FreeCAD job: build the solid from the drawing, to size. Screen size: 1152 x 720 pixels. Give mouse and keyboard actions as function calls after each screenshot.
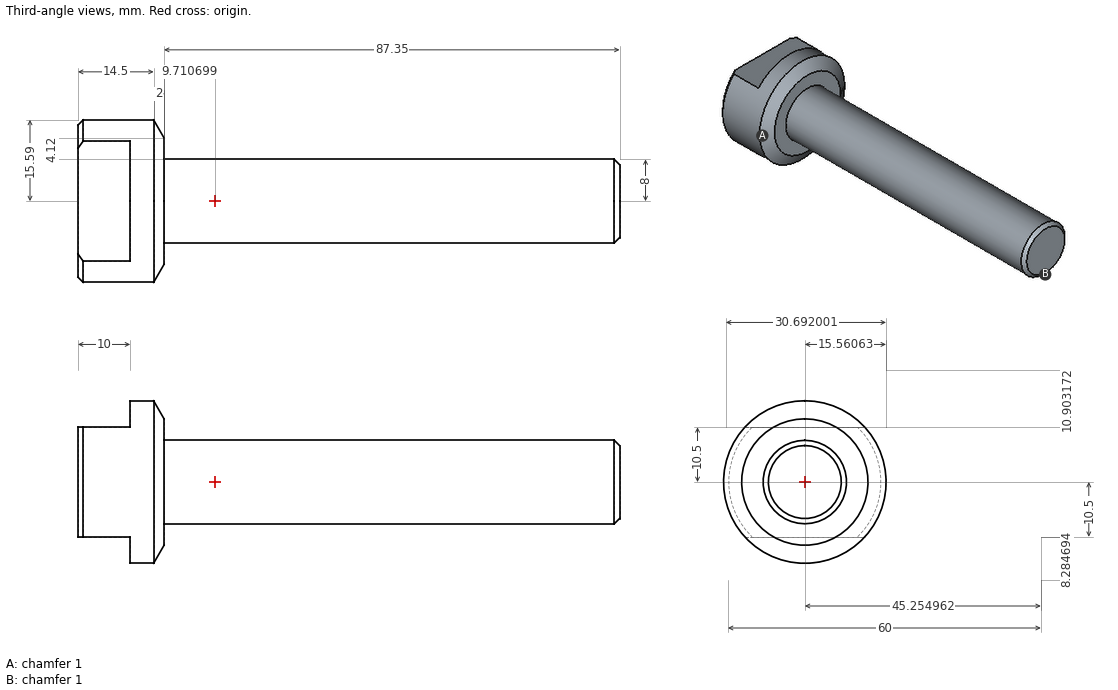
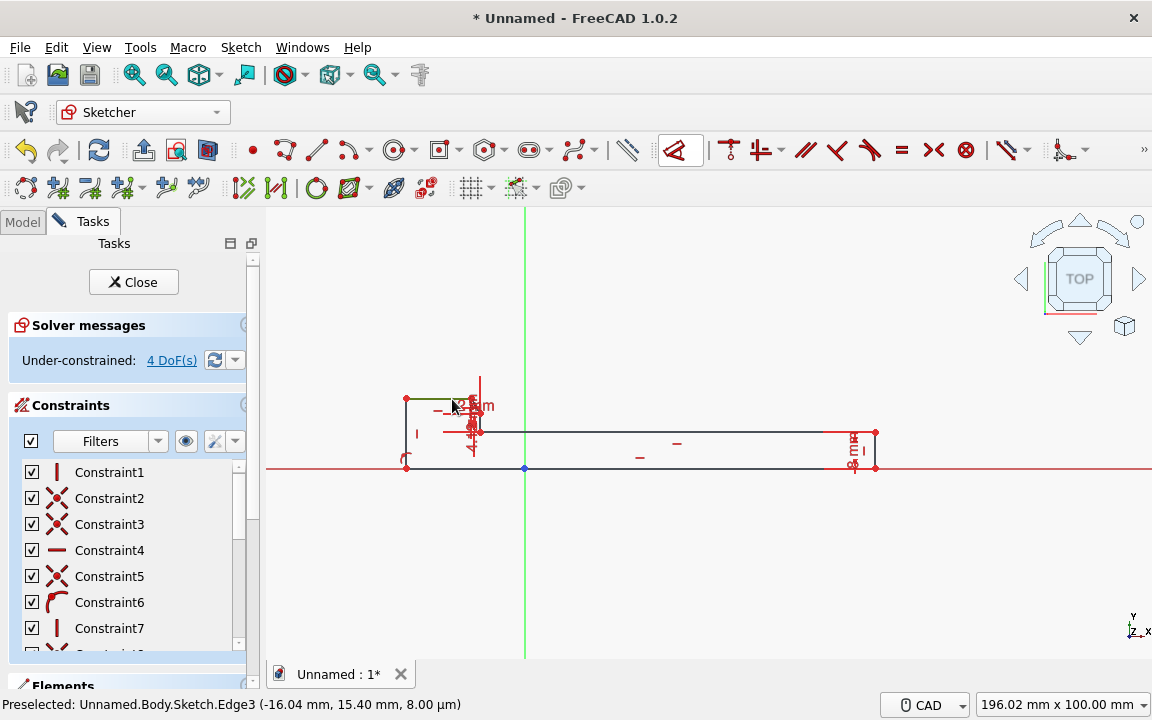
click(698, 150)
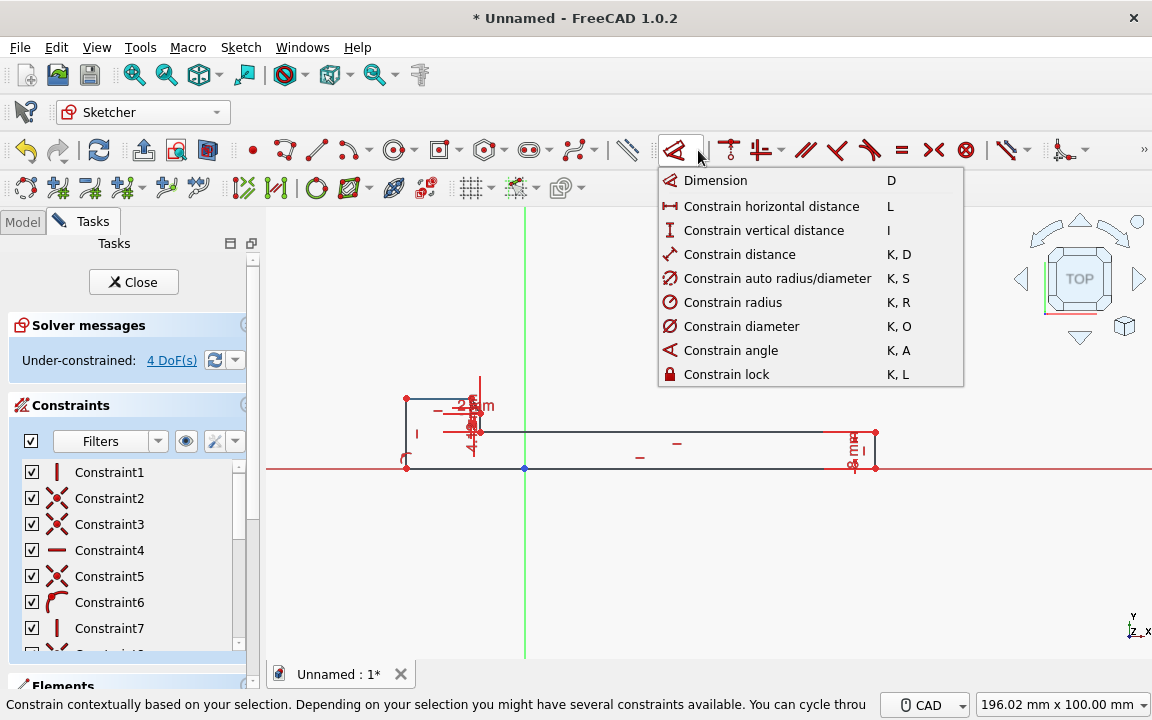
click(811, 206)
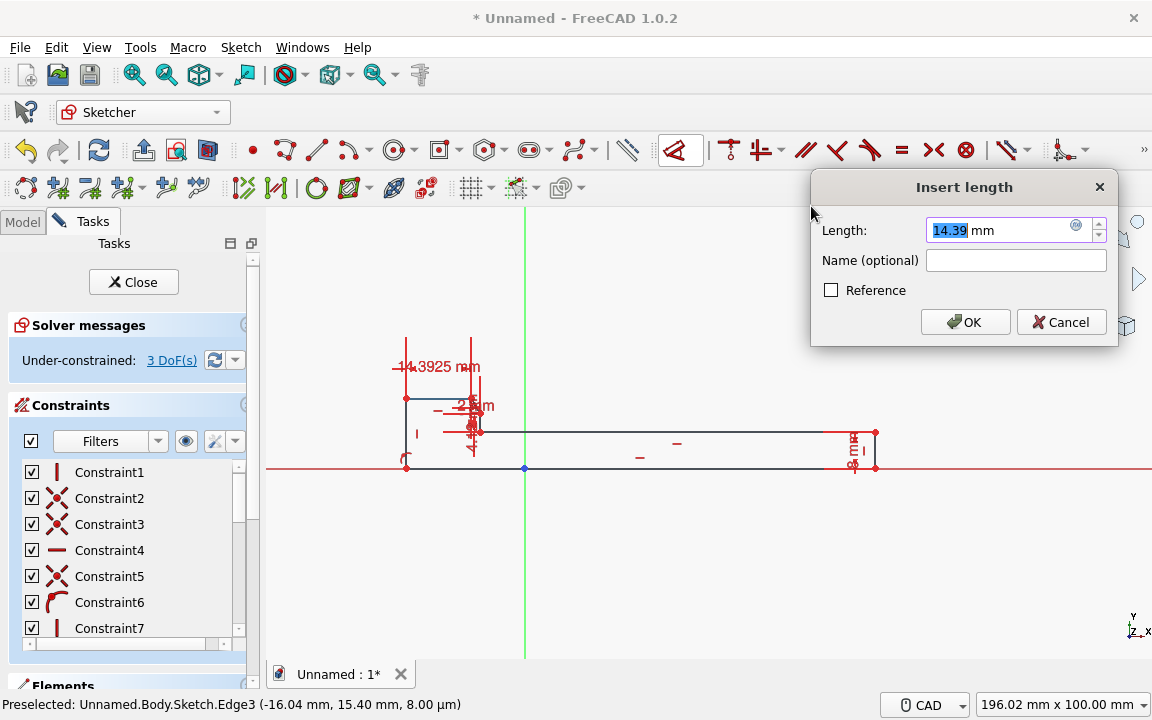
text(14.5)
key(Return)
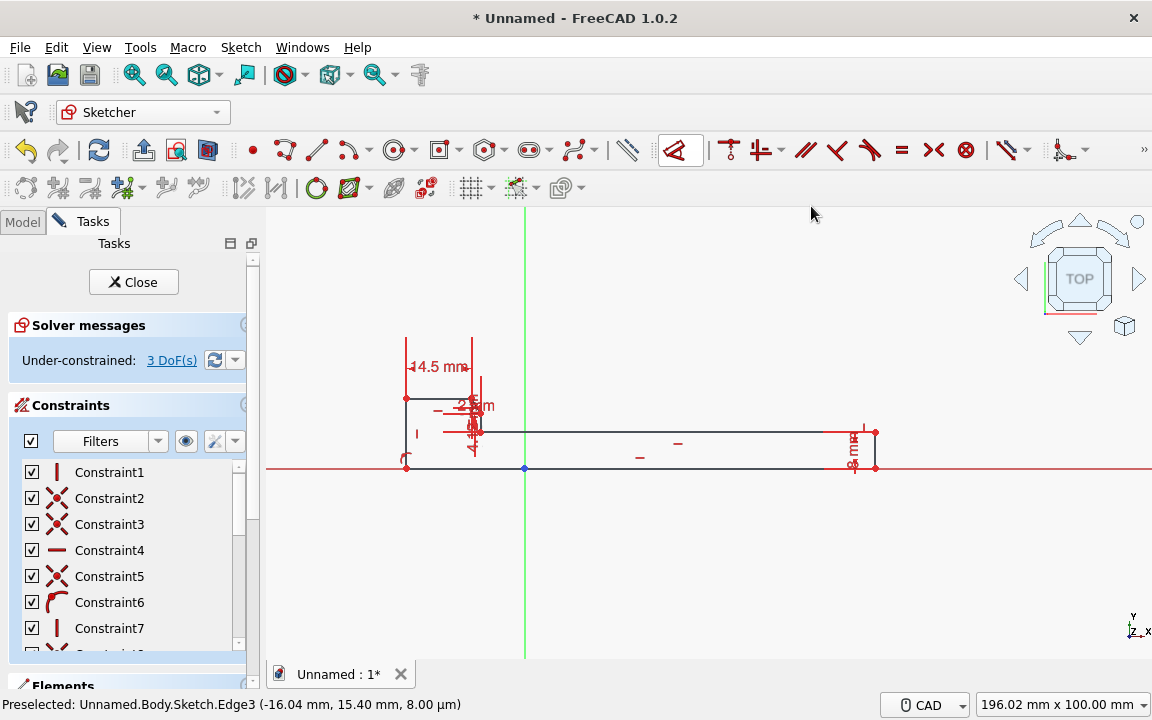
click(406, 420)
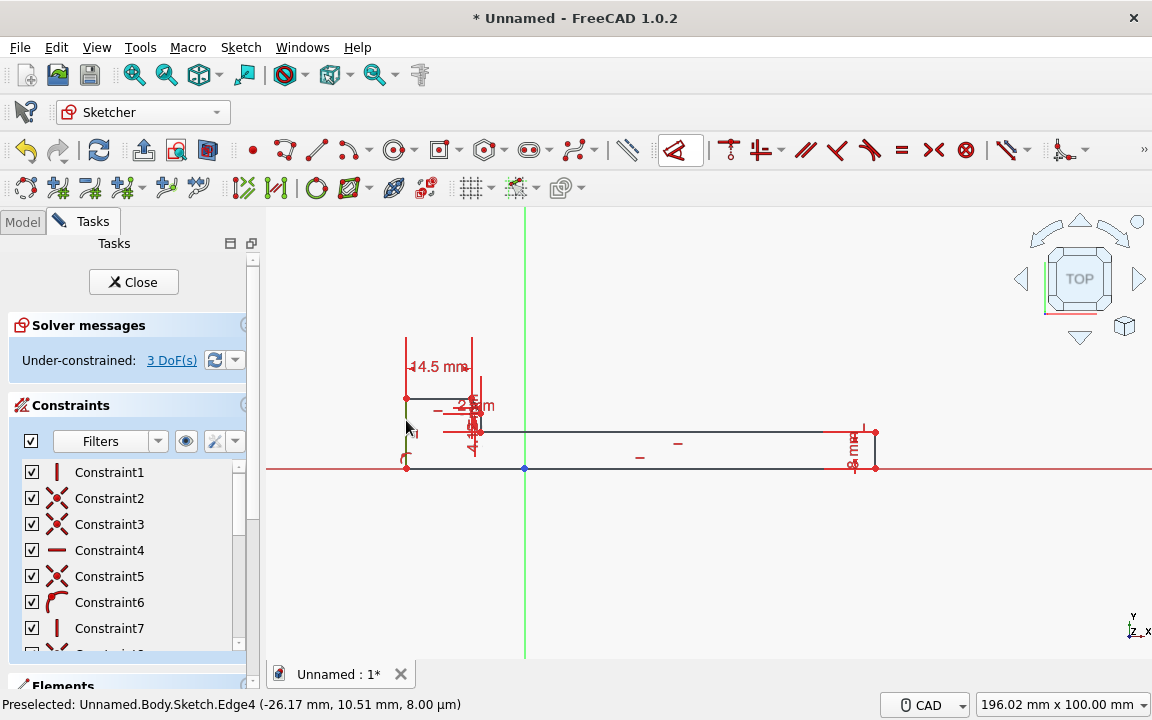
click(698, 150)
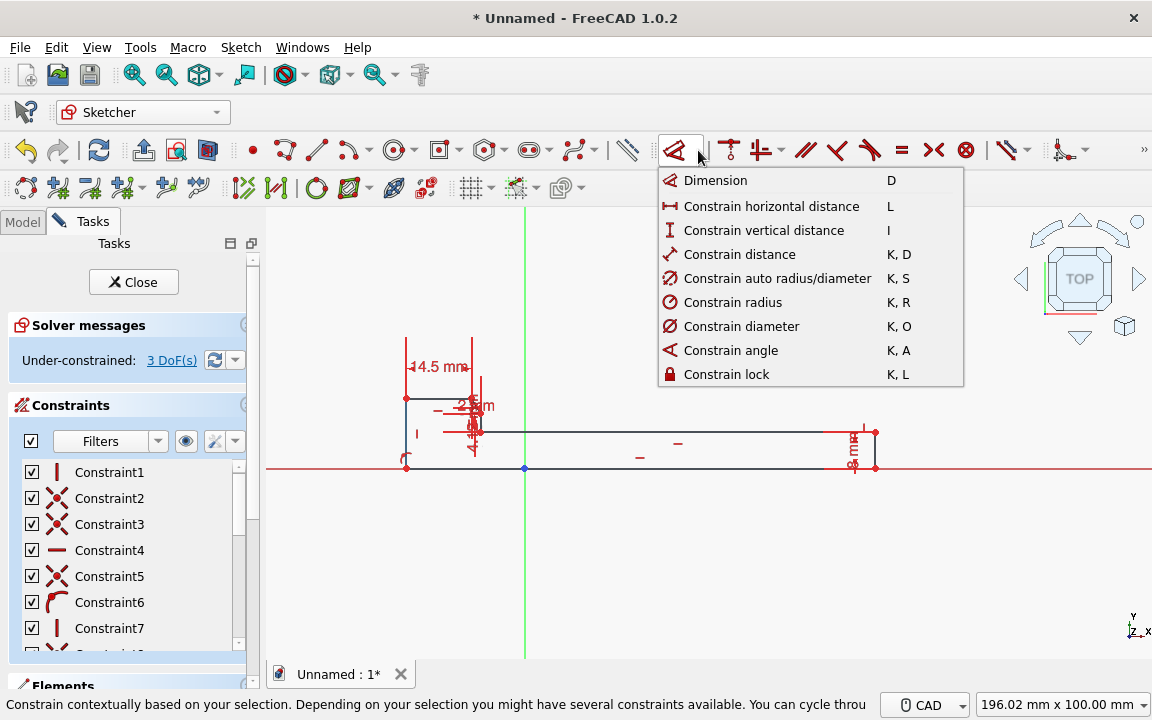
click(811, 230)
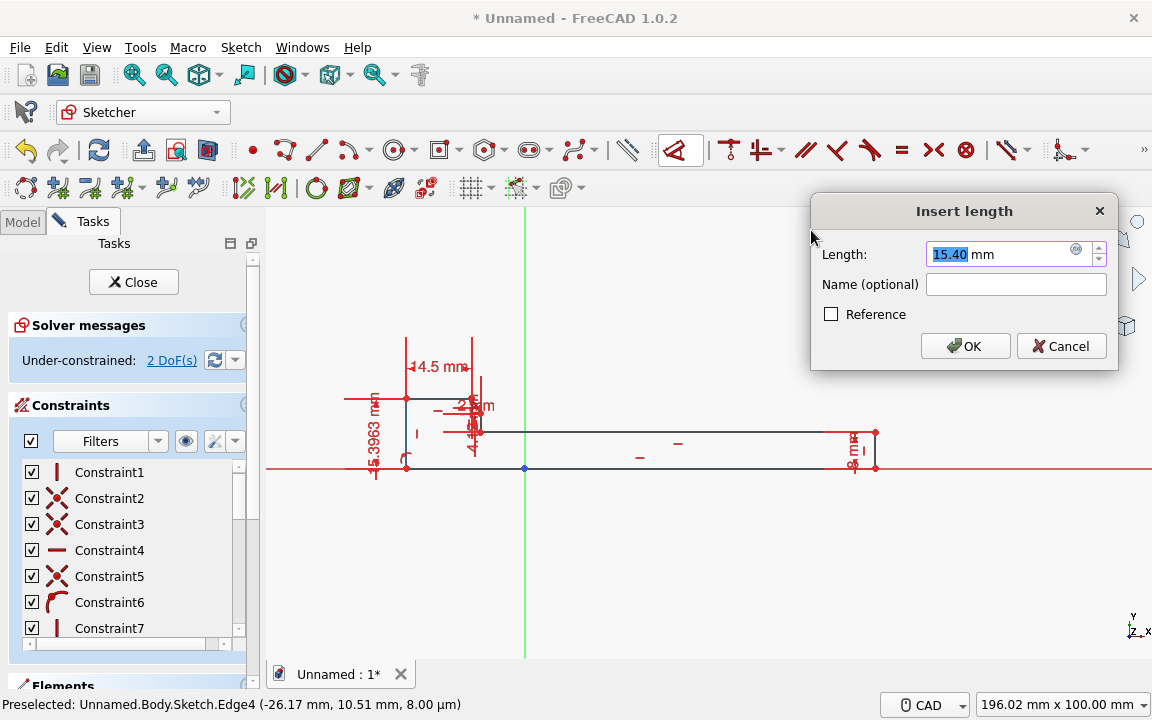
text(15.59)
key(Return)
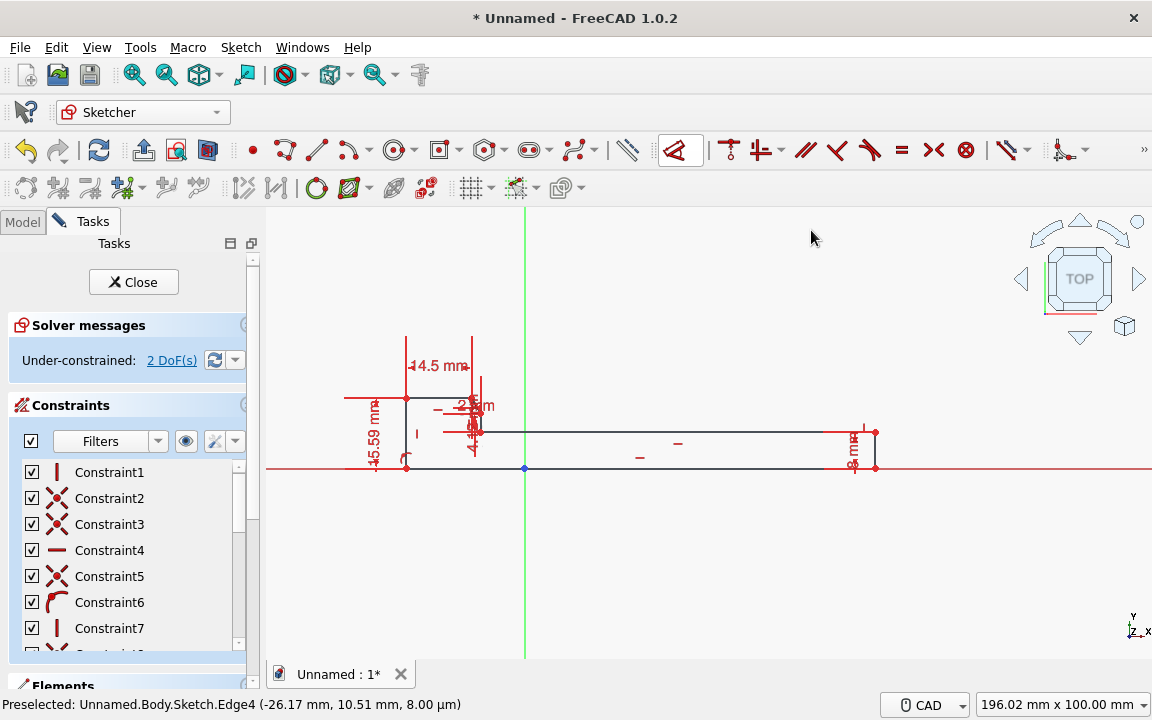
click(757, 432)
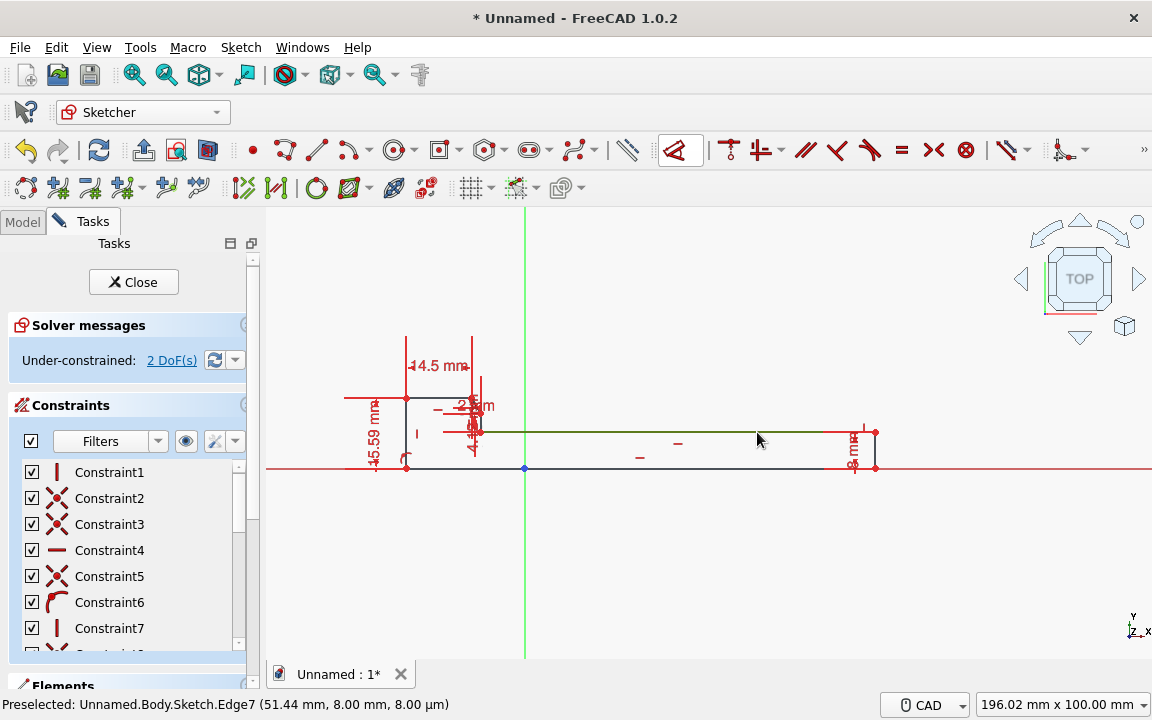
key(l)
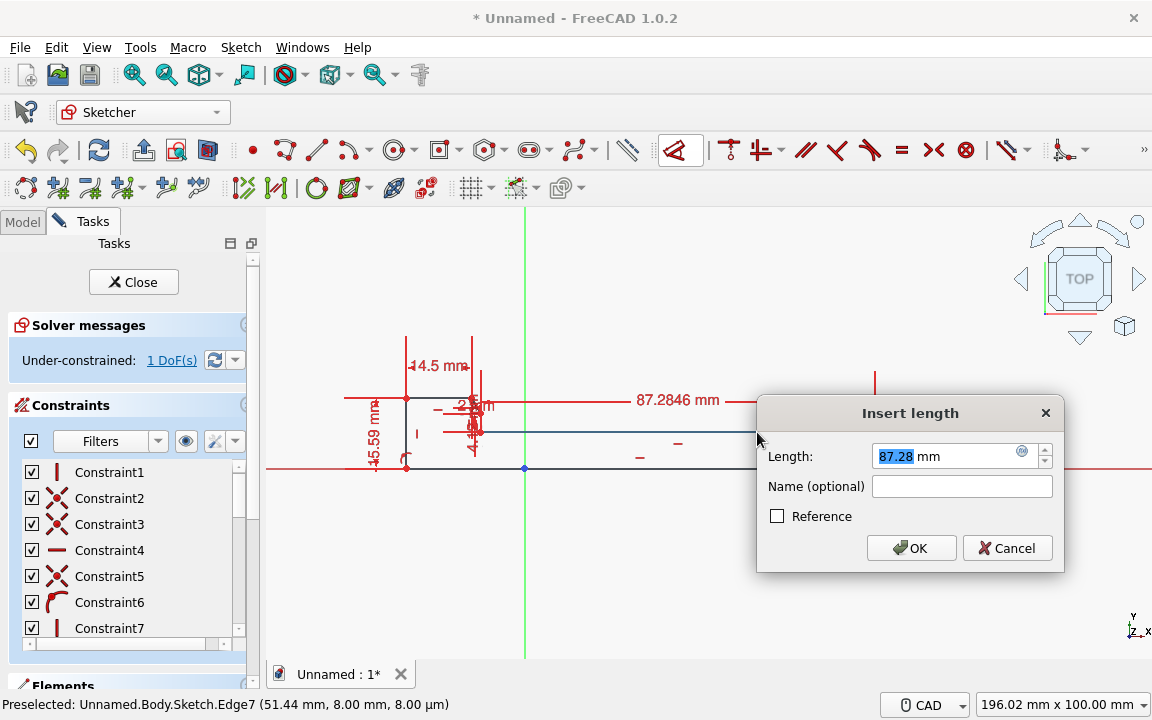
text(87.35)
key(Return)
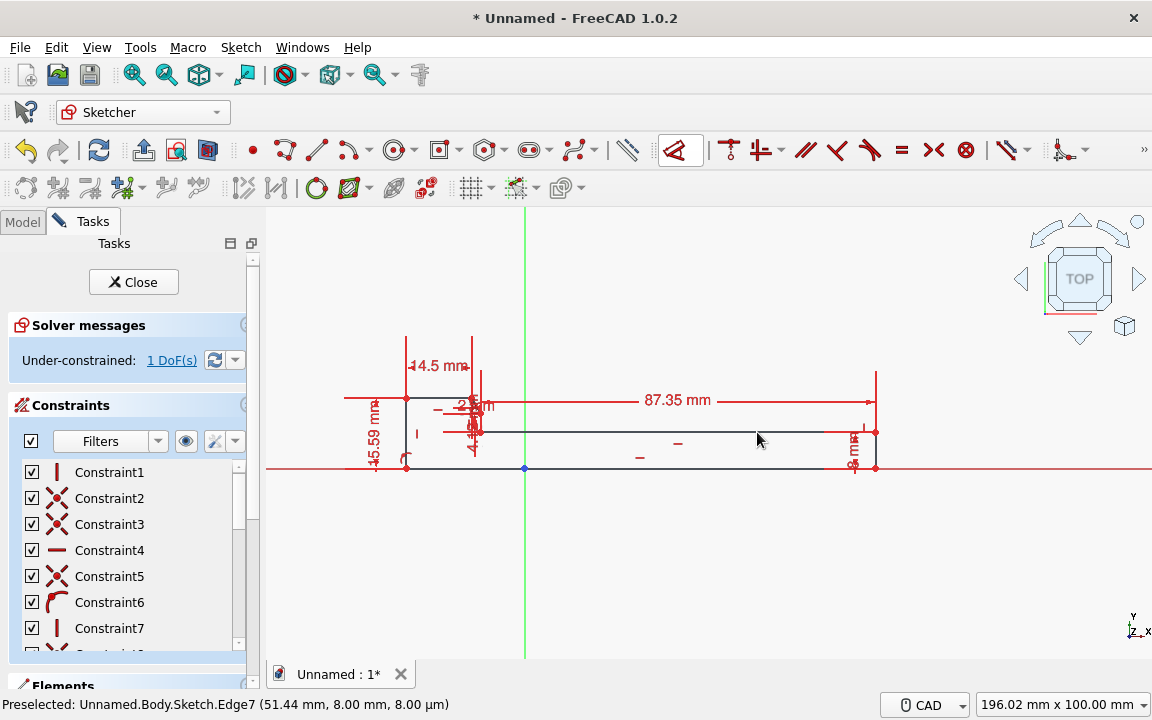
click(481, 432)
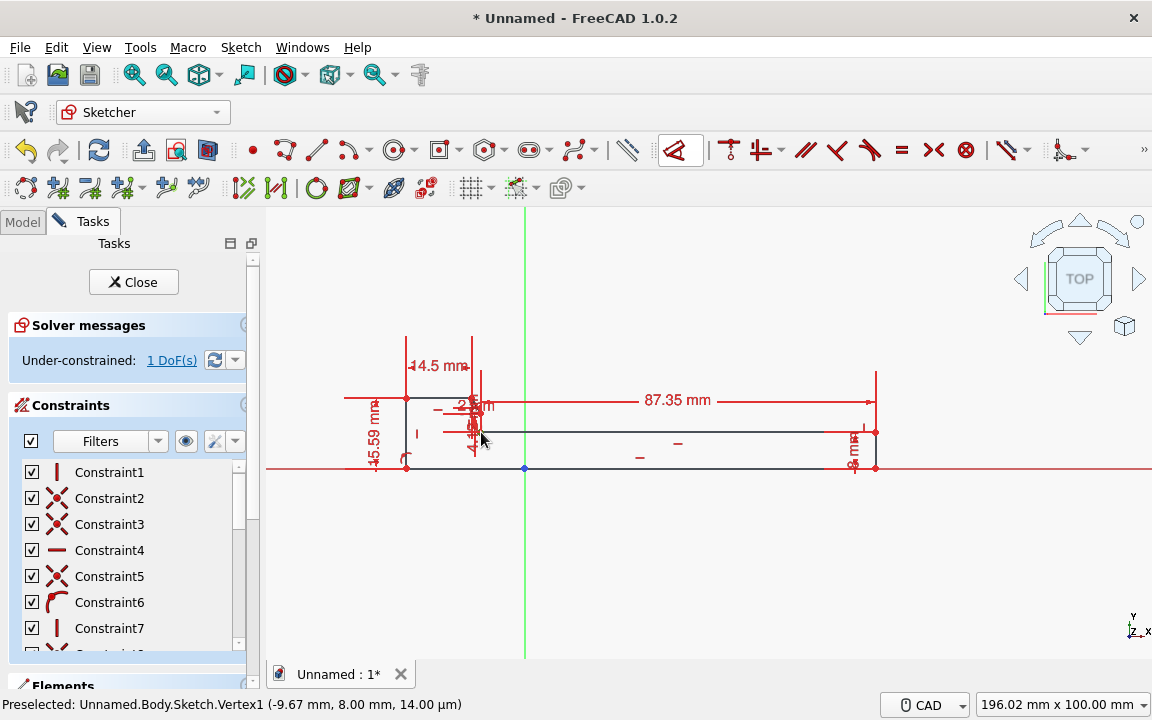
click(698, 150)